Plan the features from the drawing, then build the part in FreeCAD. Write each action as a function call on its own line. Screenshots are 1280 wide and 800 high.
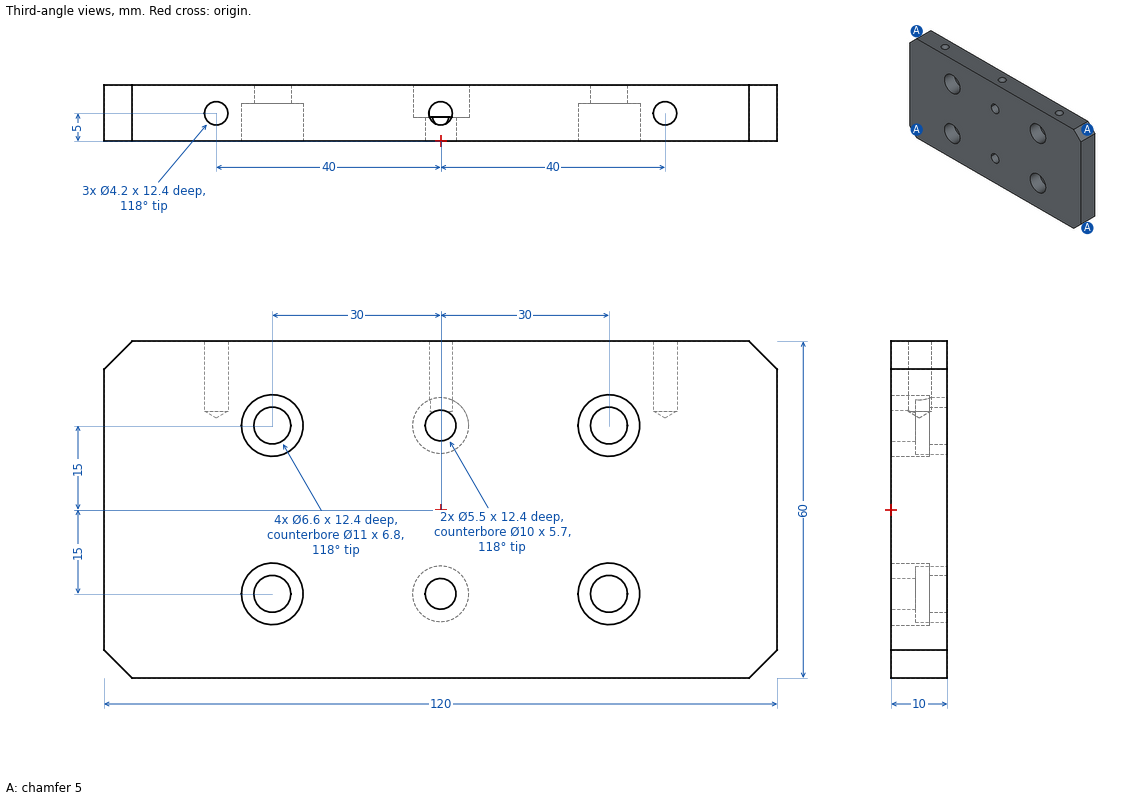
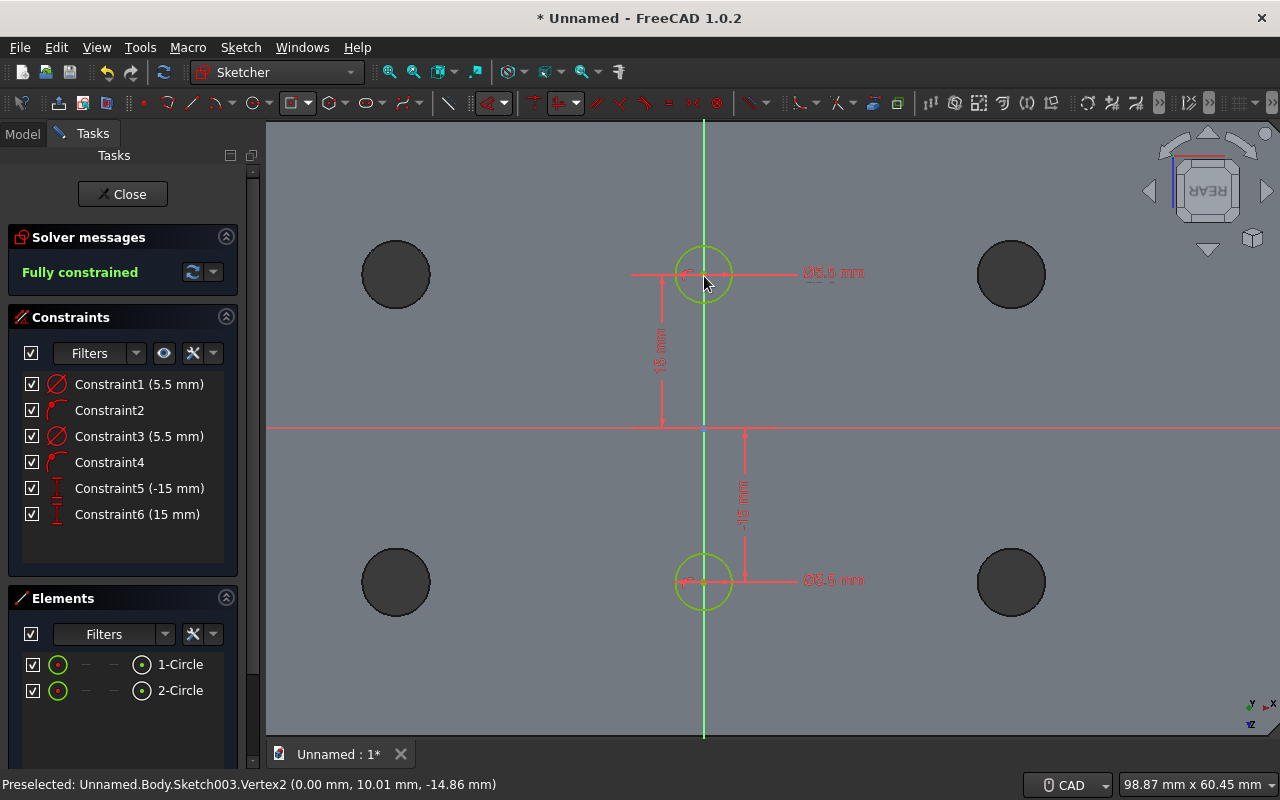
click(123, 194)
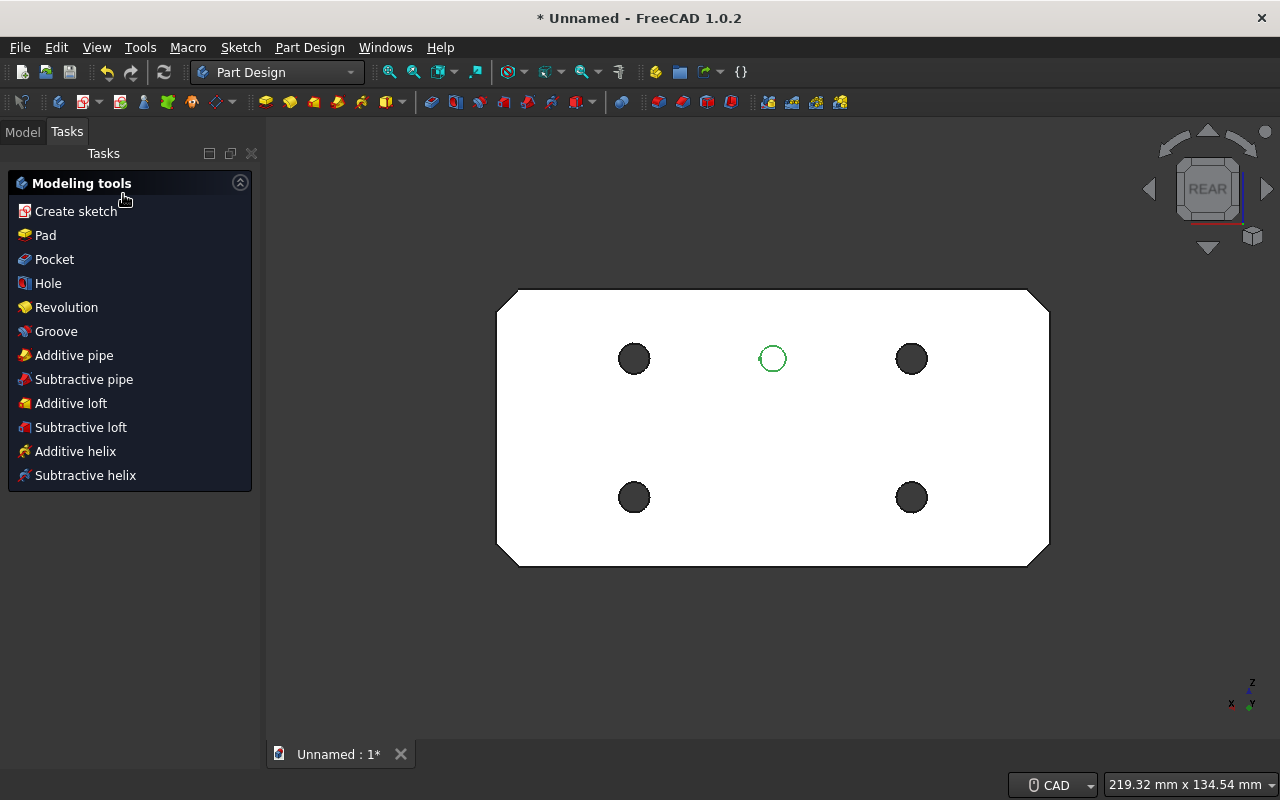
click(456, 102)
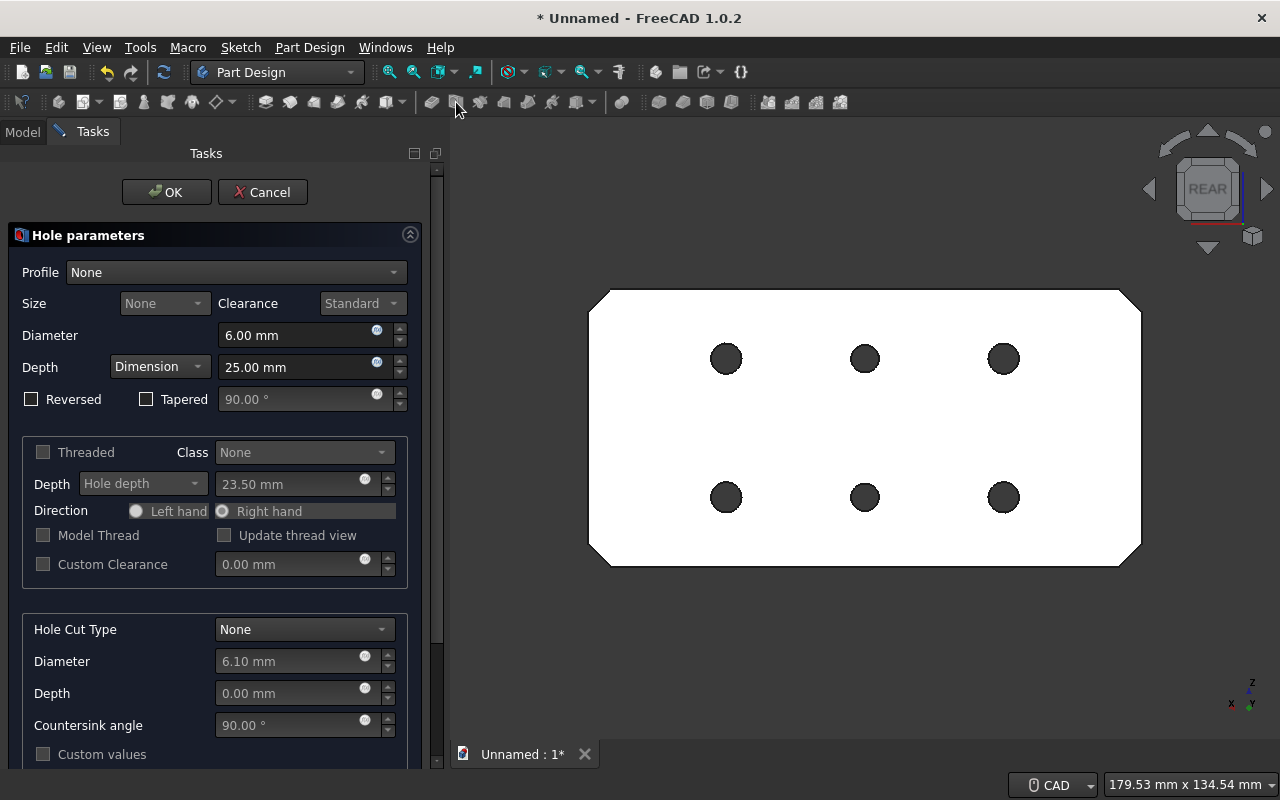
triple_click(305, 335)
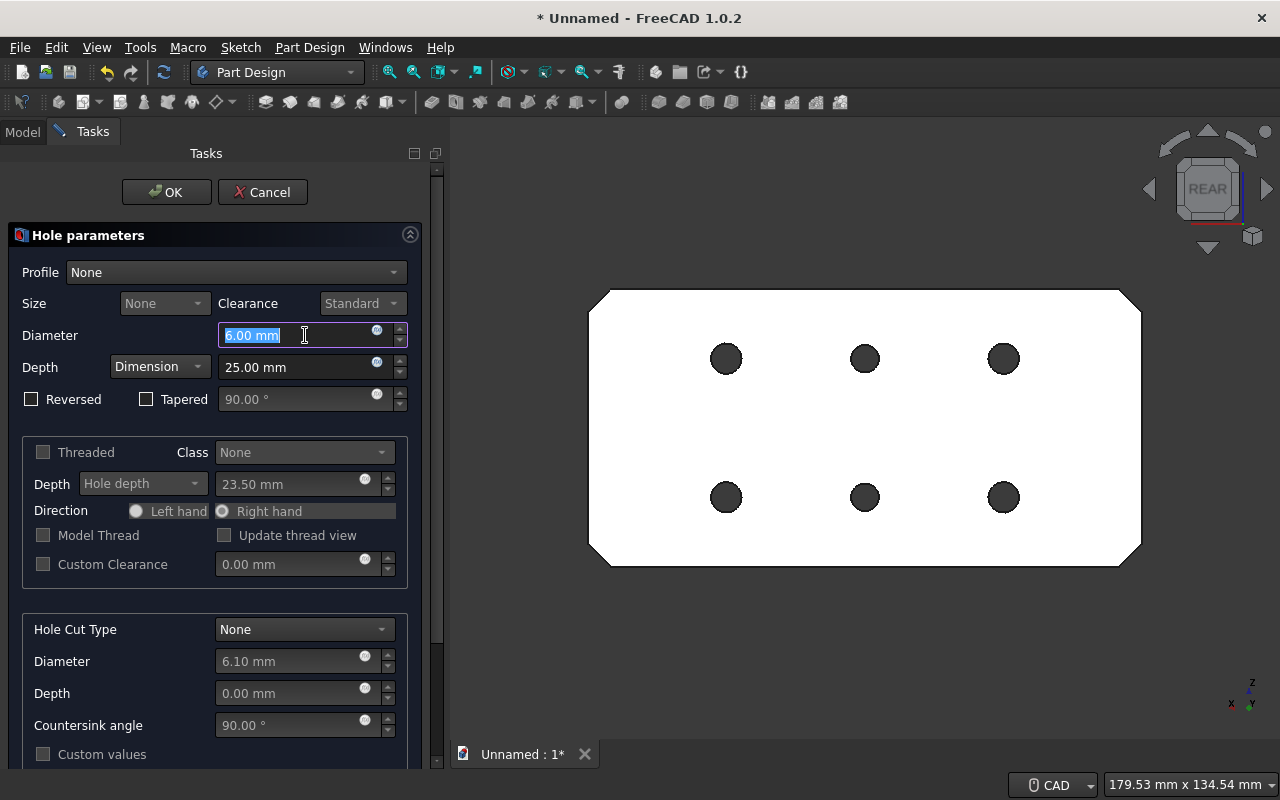
text(5.5)
key(Tab)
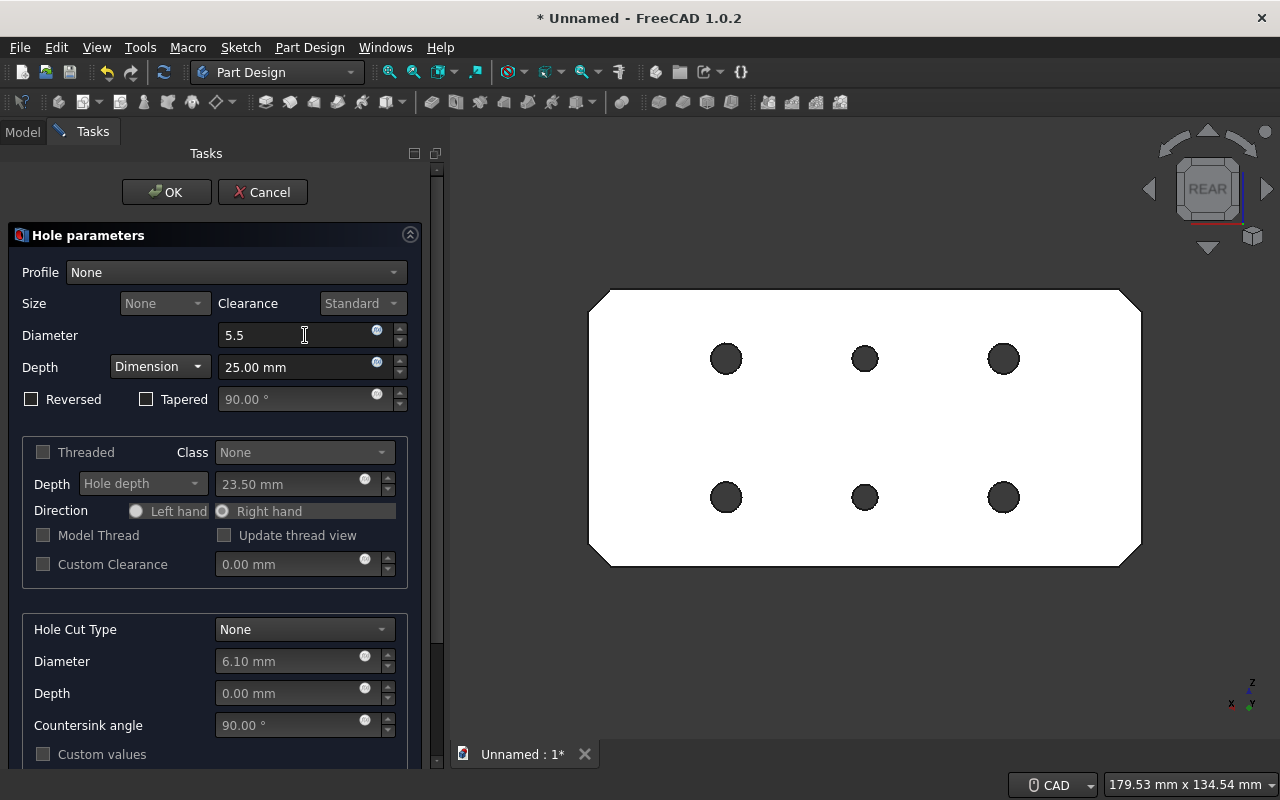
triple_click(305, 367)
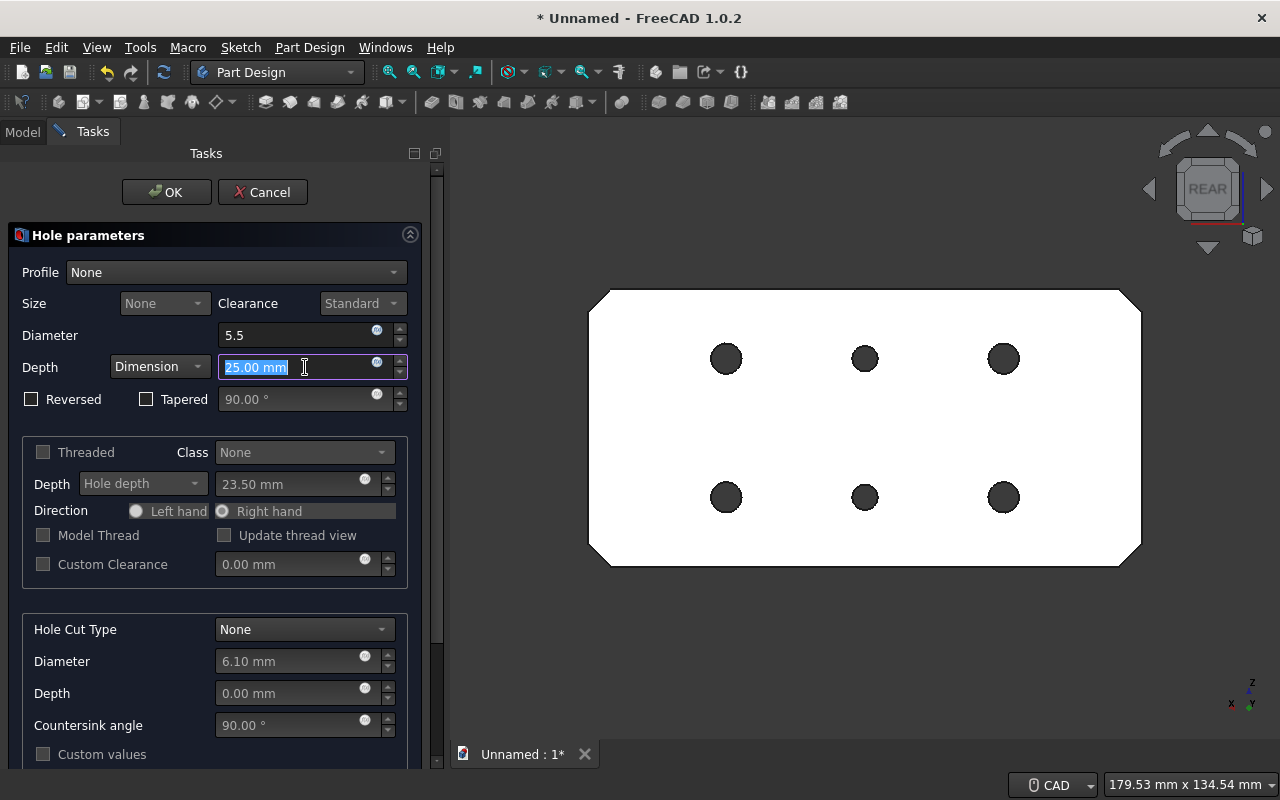
text(12.4)
key(Tab)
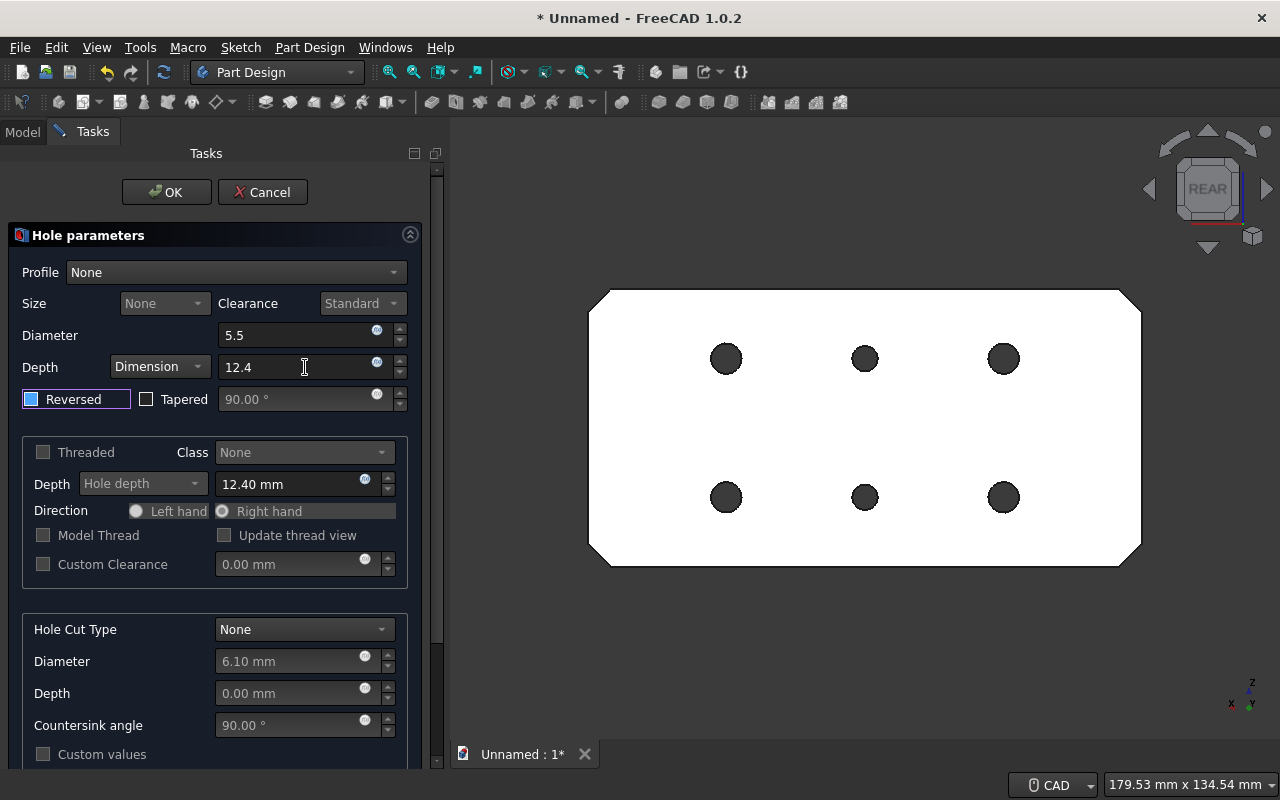
click(306, 630)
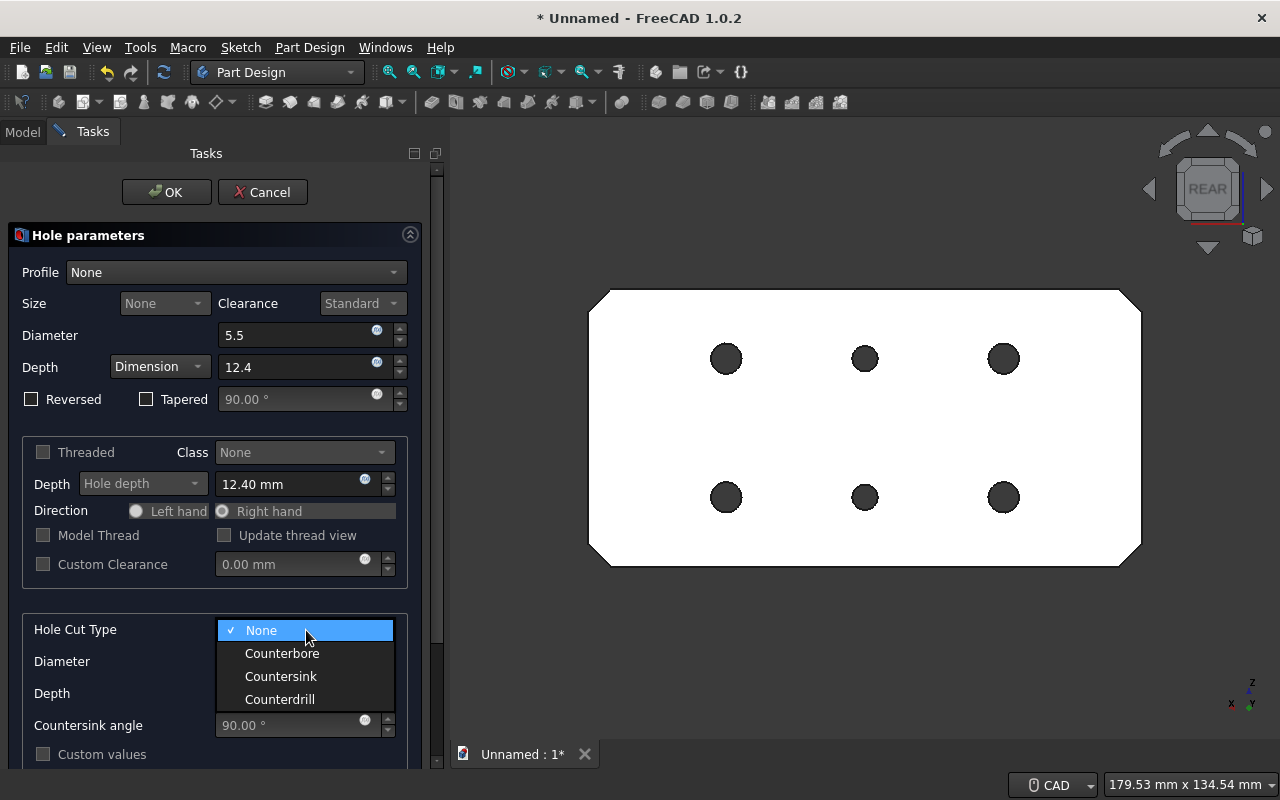
click(304, 654)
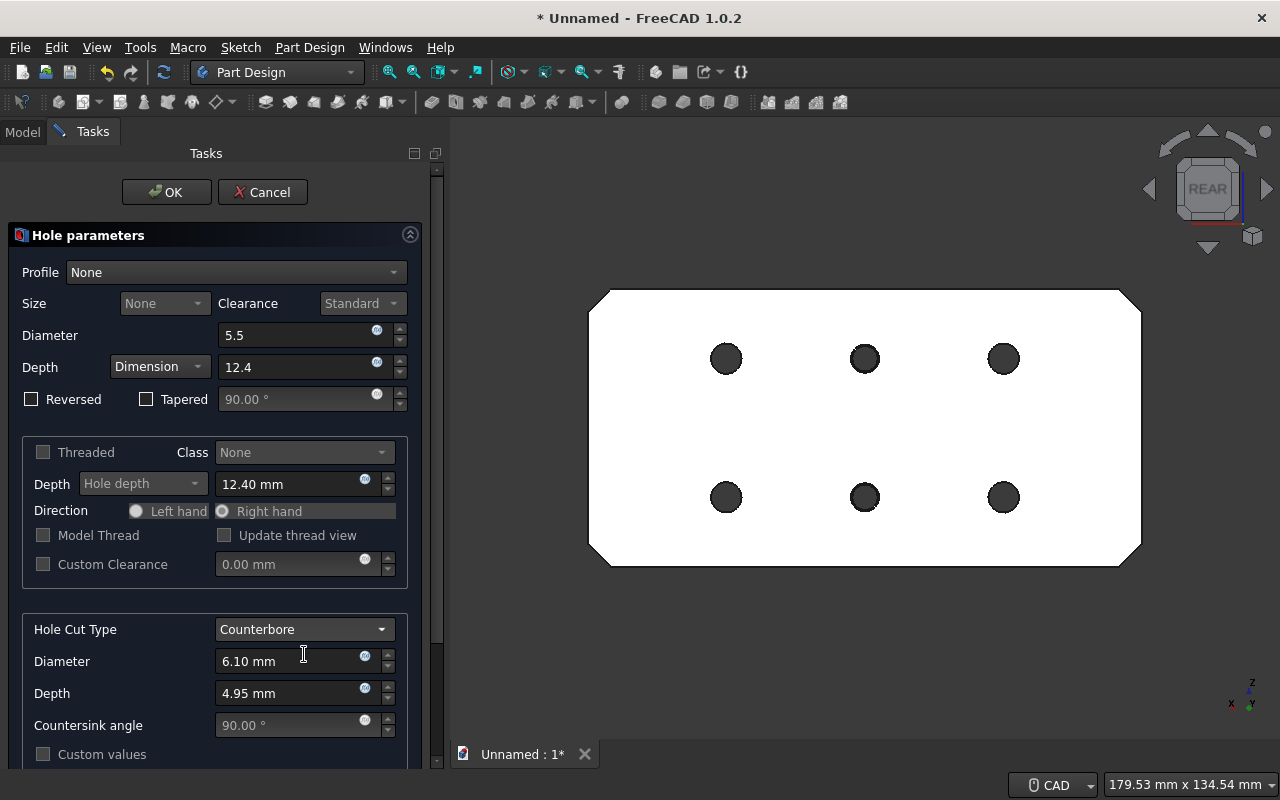
triple_click(298, 661)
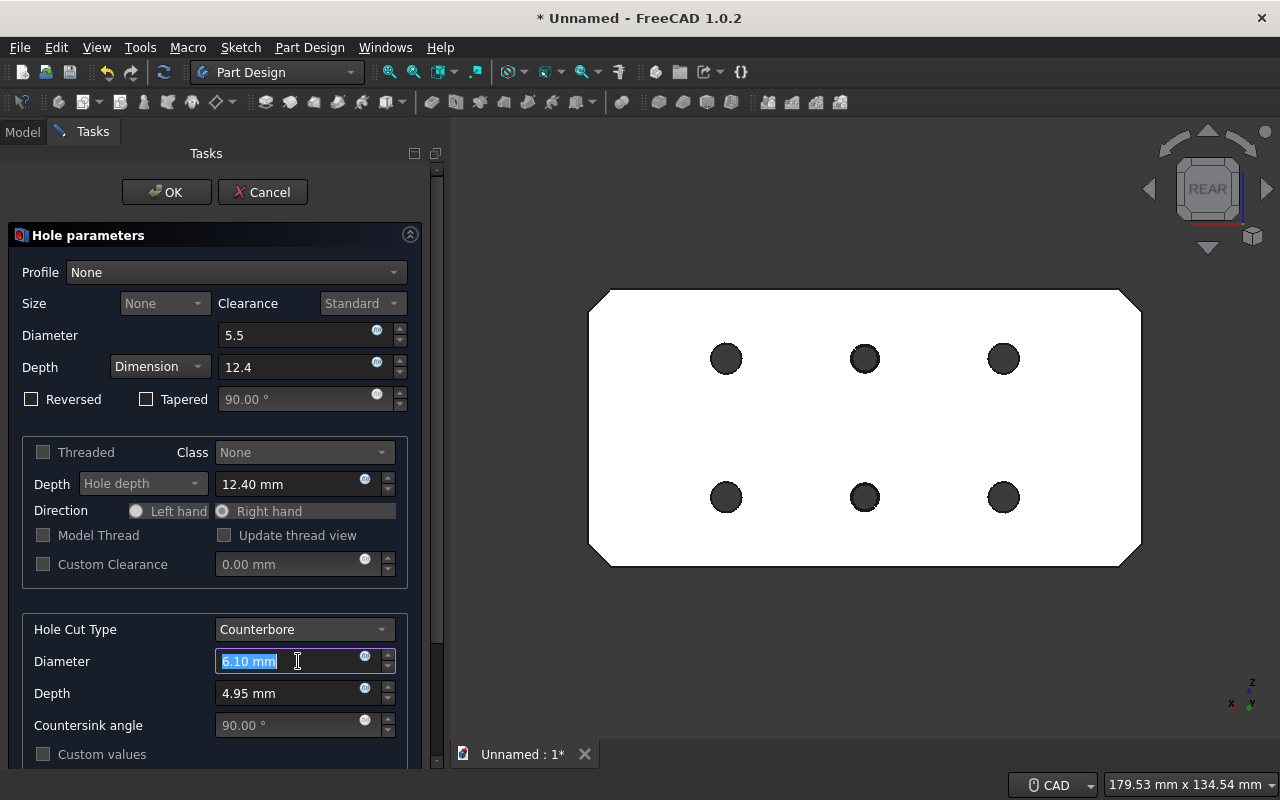
text(10)
key(Tab)